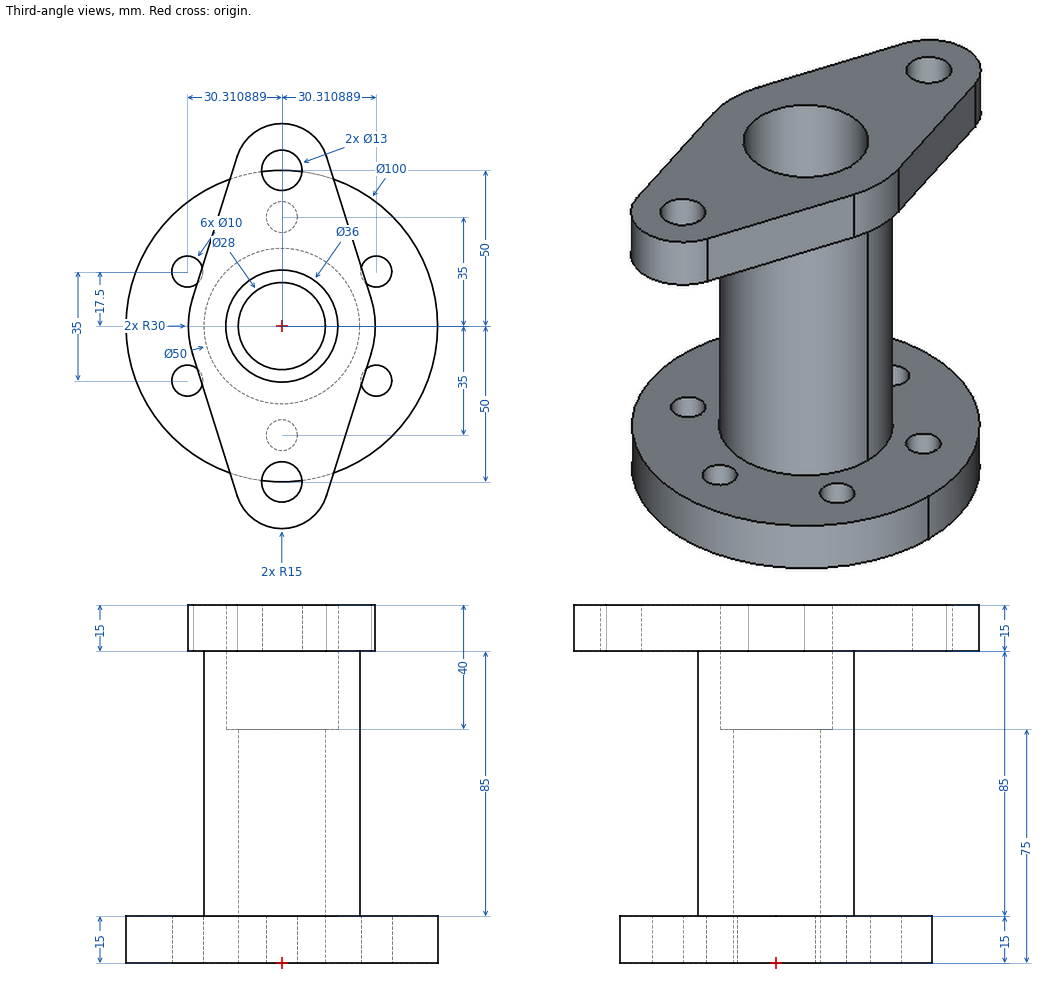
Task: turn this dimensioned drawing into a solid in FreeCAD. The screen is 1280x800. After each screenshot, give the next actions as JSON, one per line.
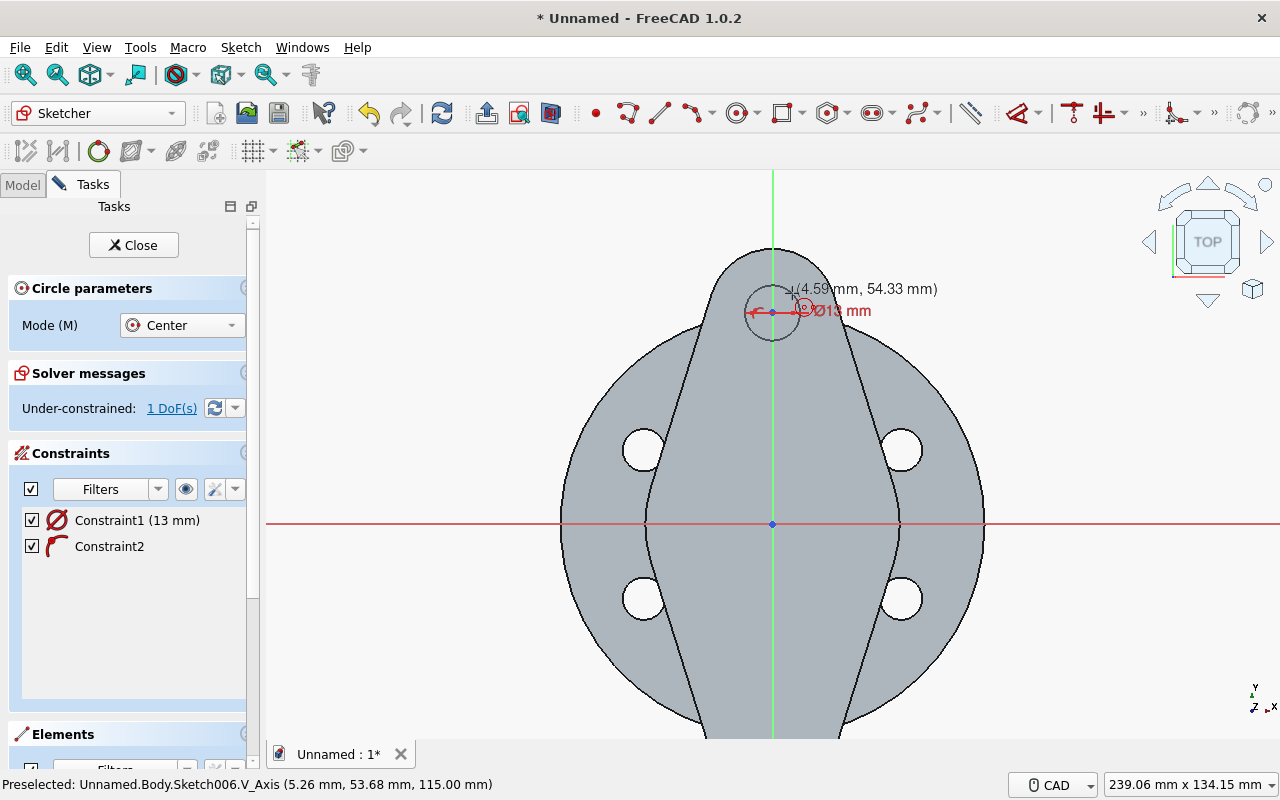
{"action": "scroll", "coordinate": [397, 198], "scroll_direction": "down", "scroll_amount": 1}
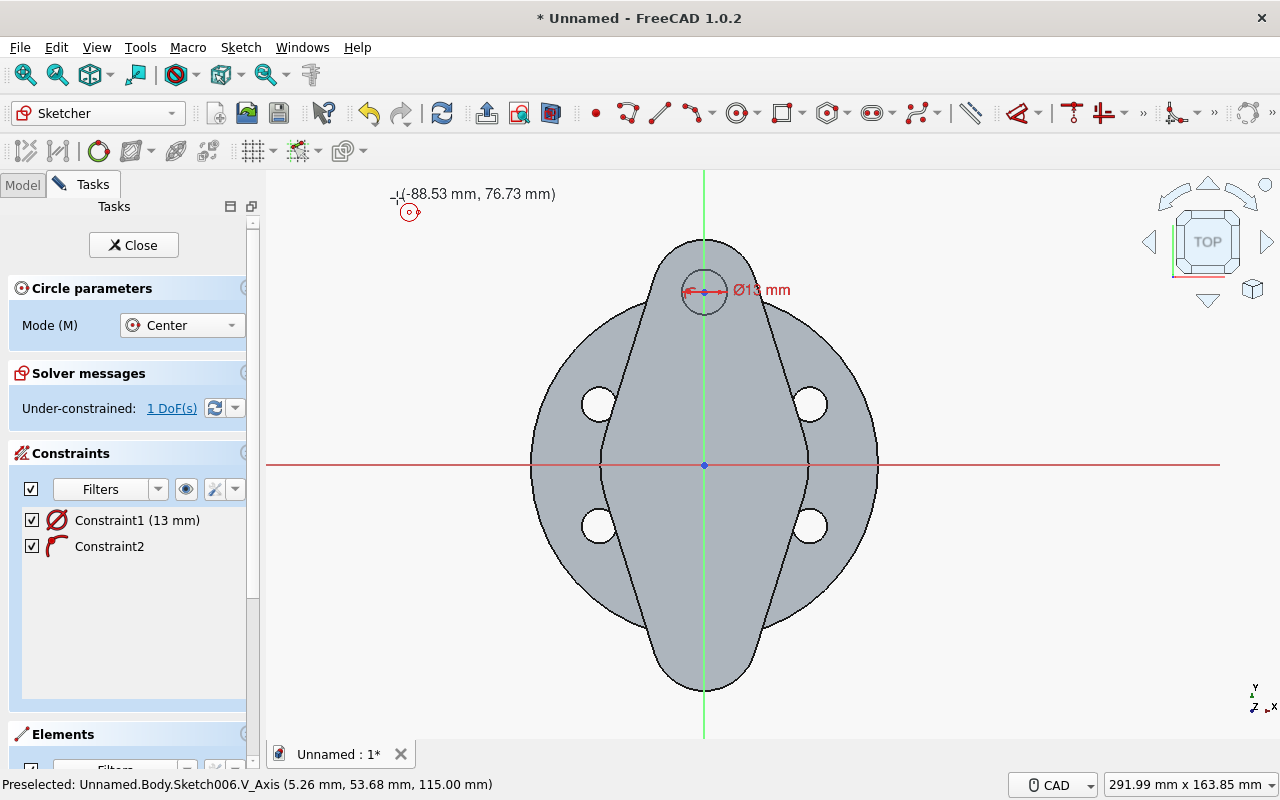
{"action": "left_click", "coordinate": [704, 639]}
{"action": "mouse_move", "coordinate": [720, 623]}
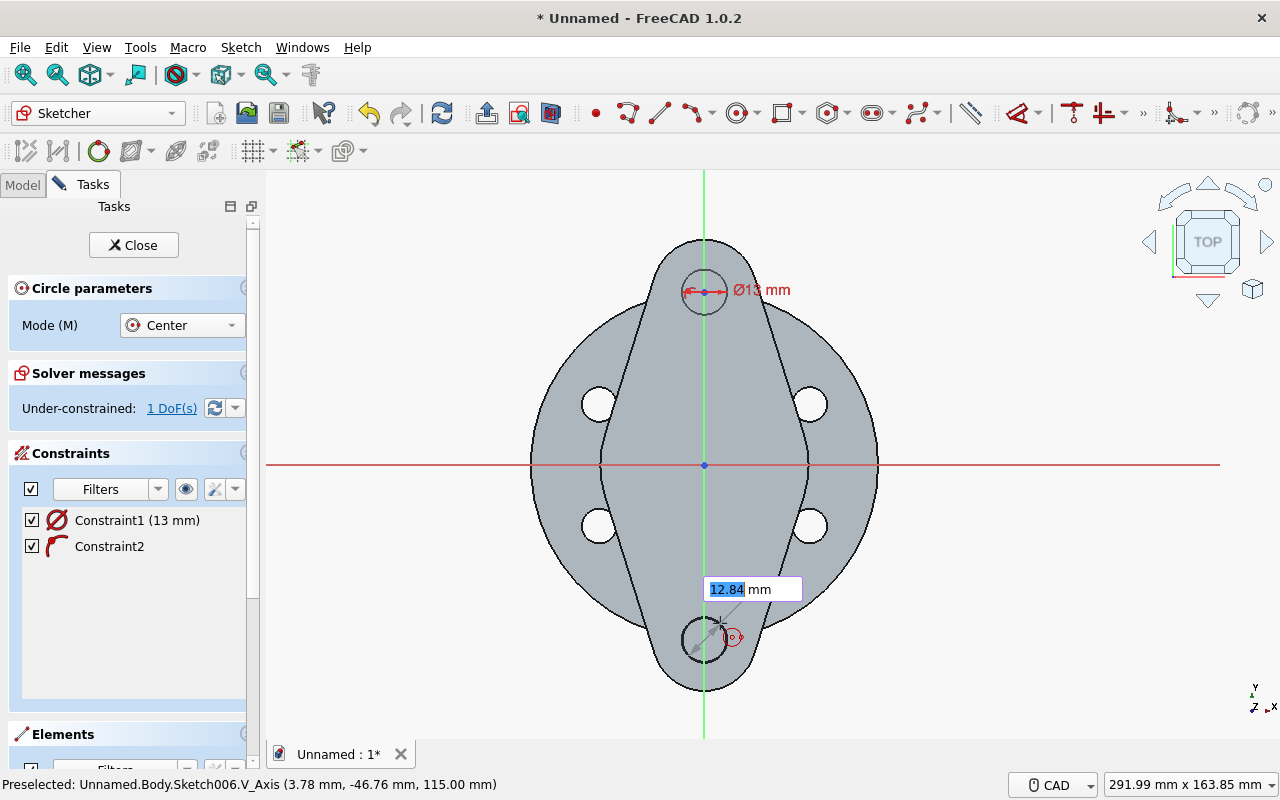
{"action": "type", "text": "13"}
{"action": "key", "text": "Return"}
{"action": "key", "text": "Escape"}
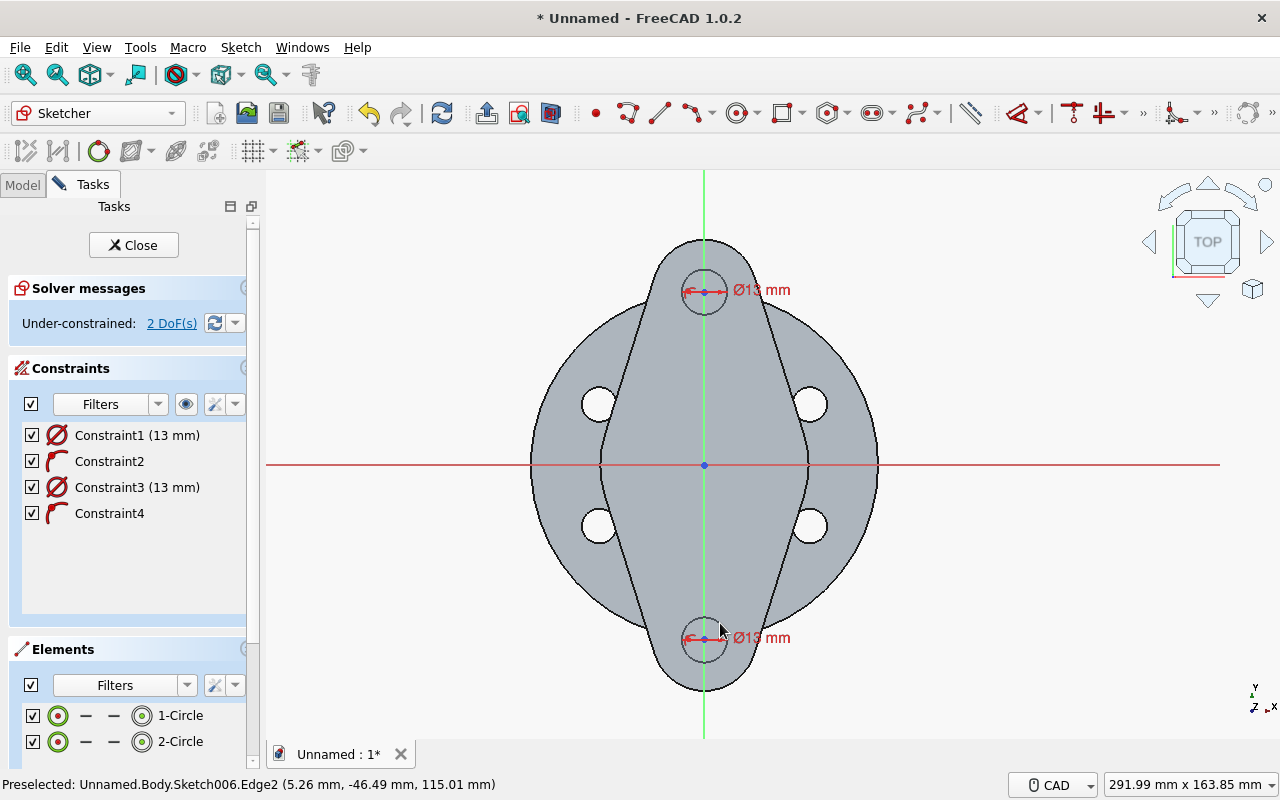
{"action": "left_click", "coordinate": [704, 292]}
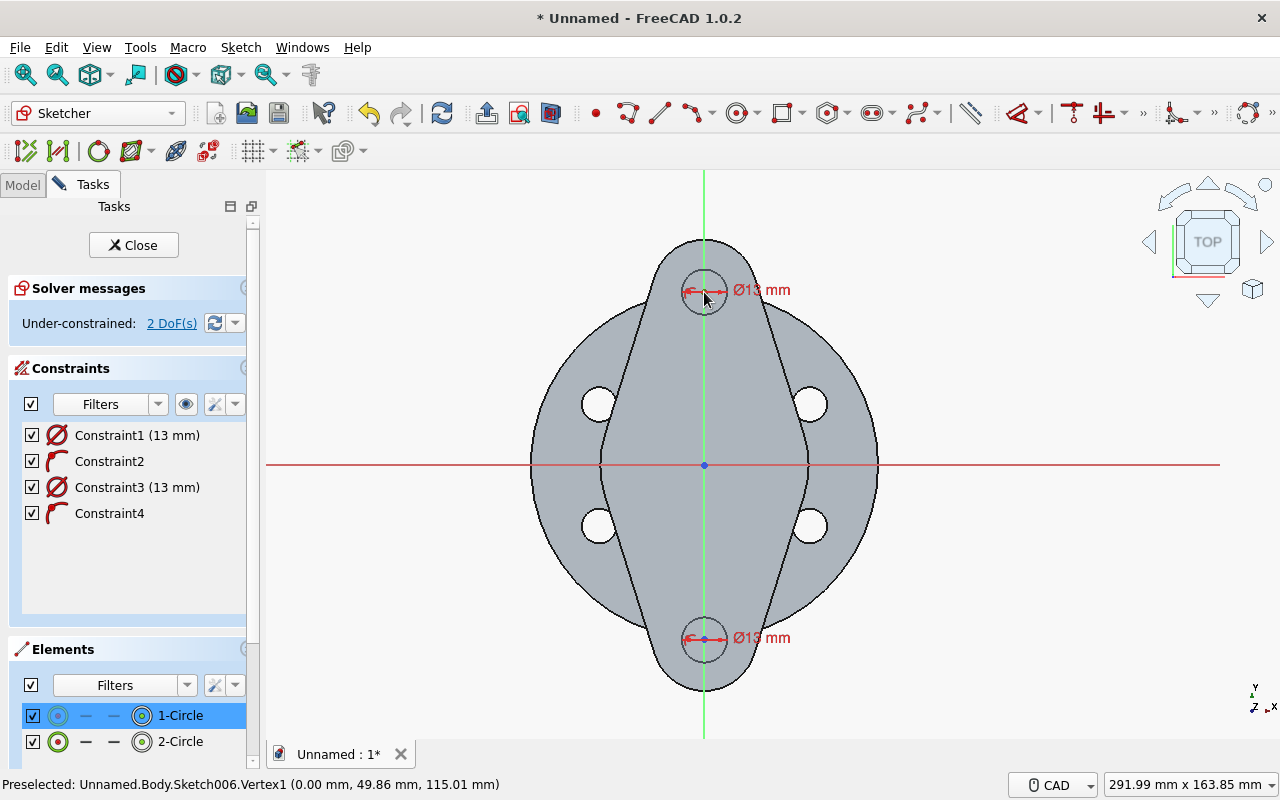
{"action": "key", "text": "i"}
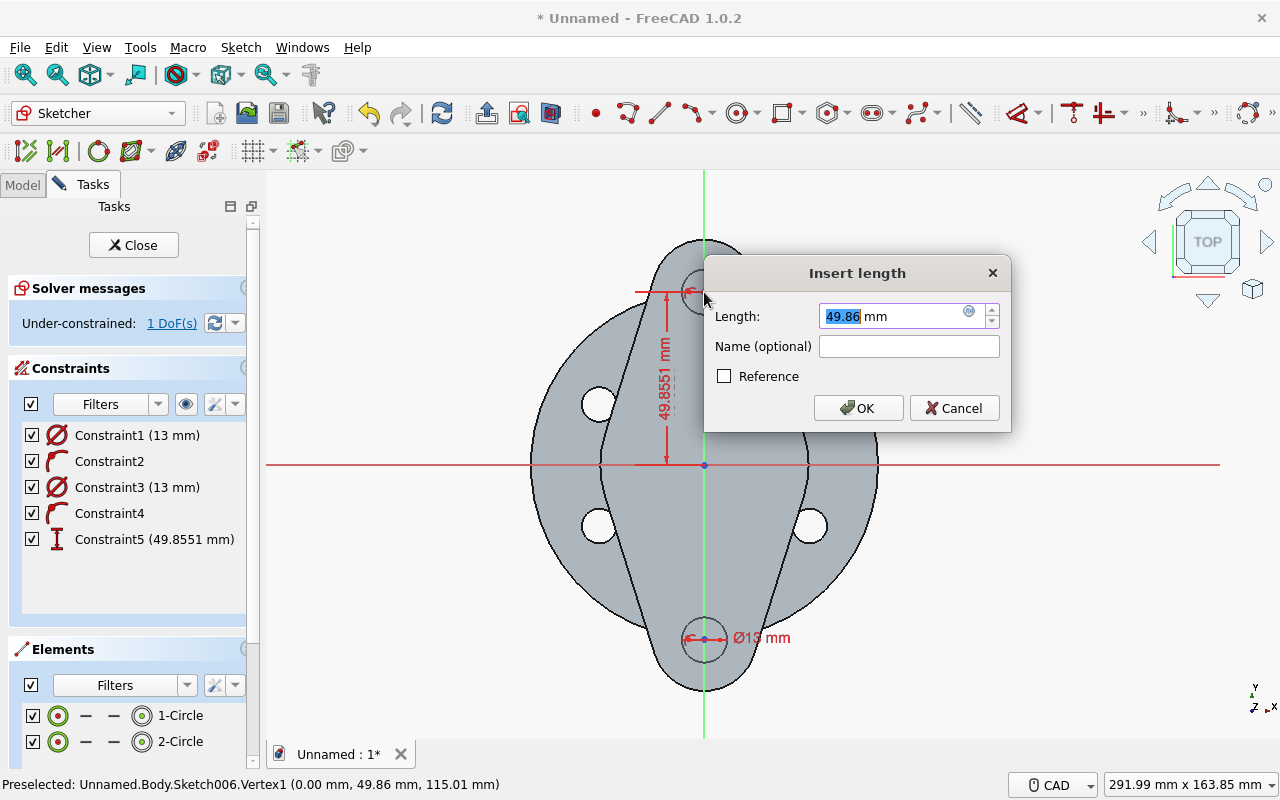
{"action": "type", "text": "50"}
{"action": "key", "text": "Return"}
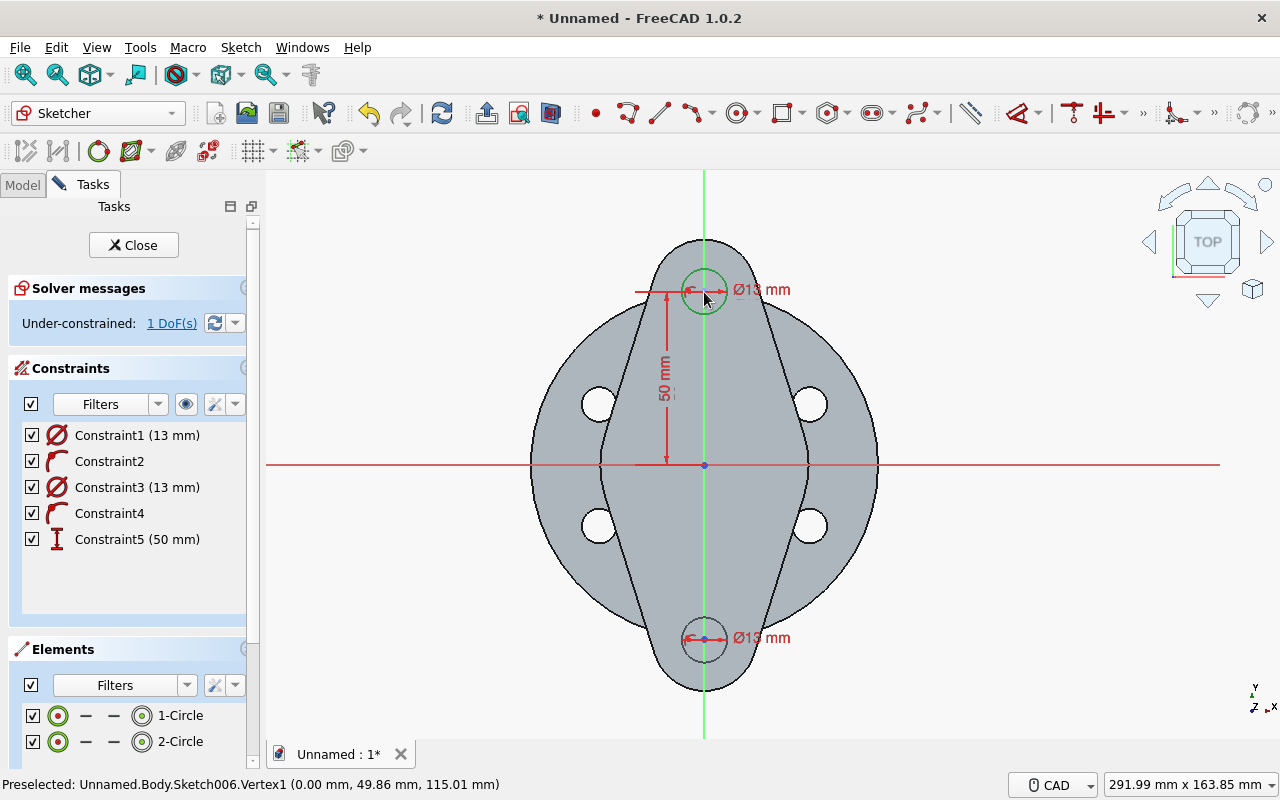
{"action": "left_click", "coordinate": [704, 640]}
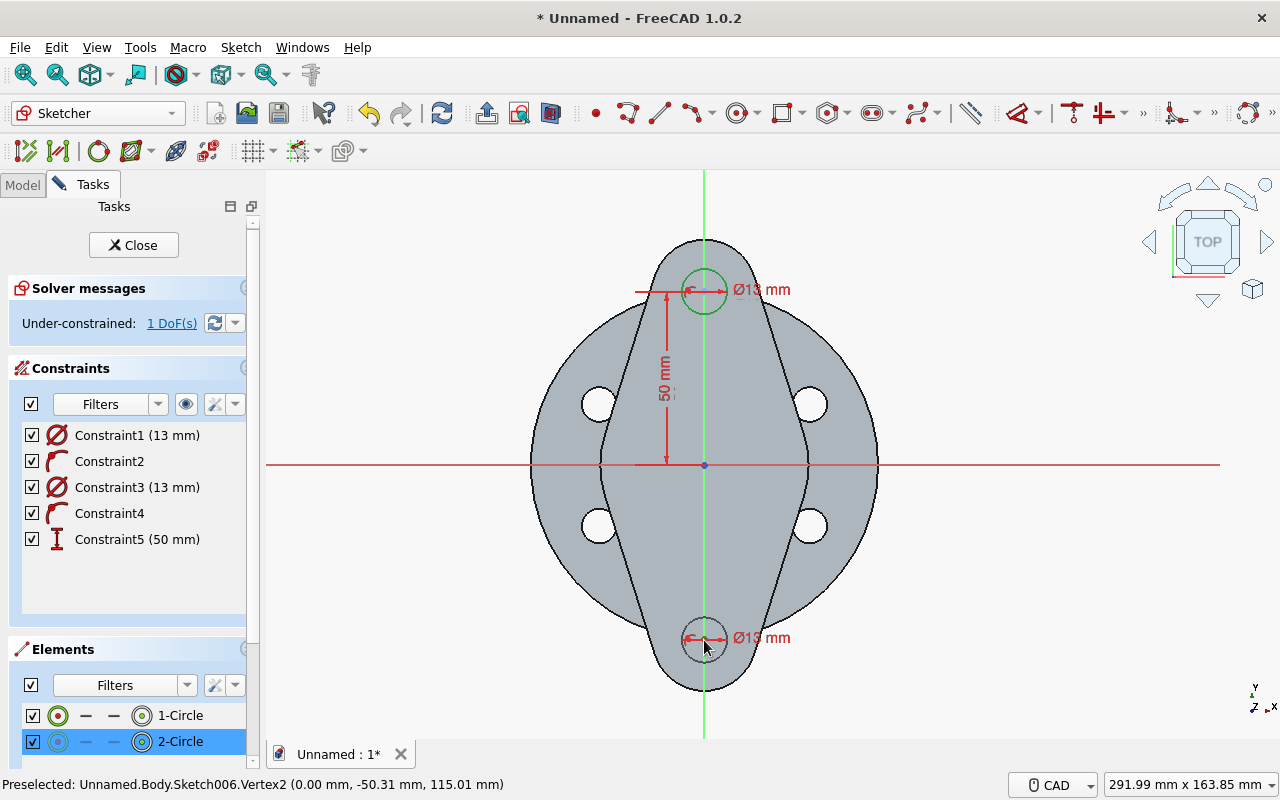
{"action": "key", "text": "i"}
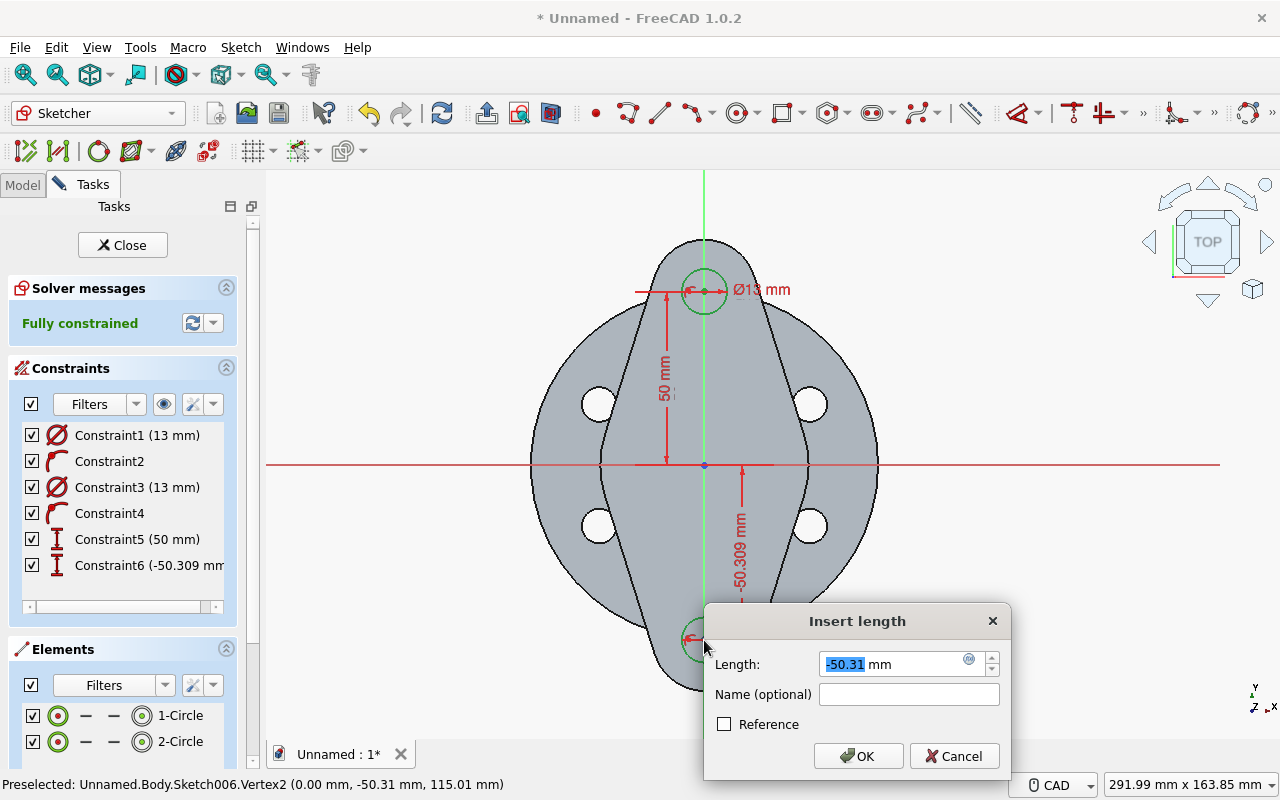
{"action": "type", "text": "-50"}
{"action": "key", "text": "Return"}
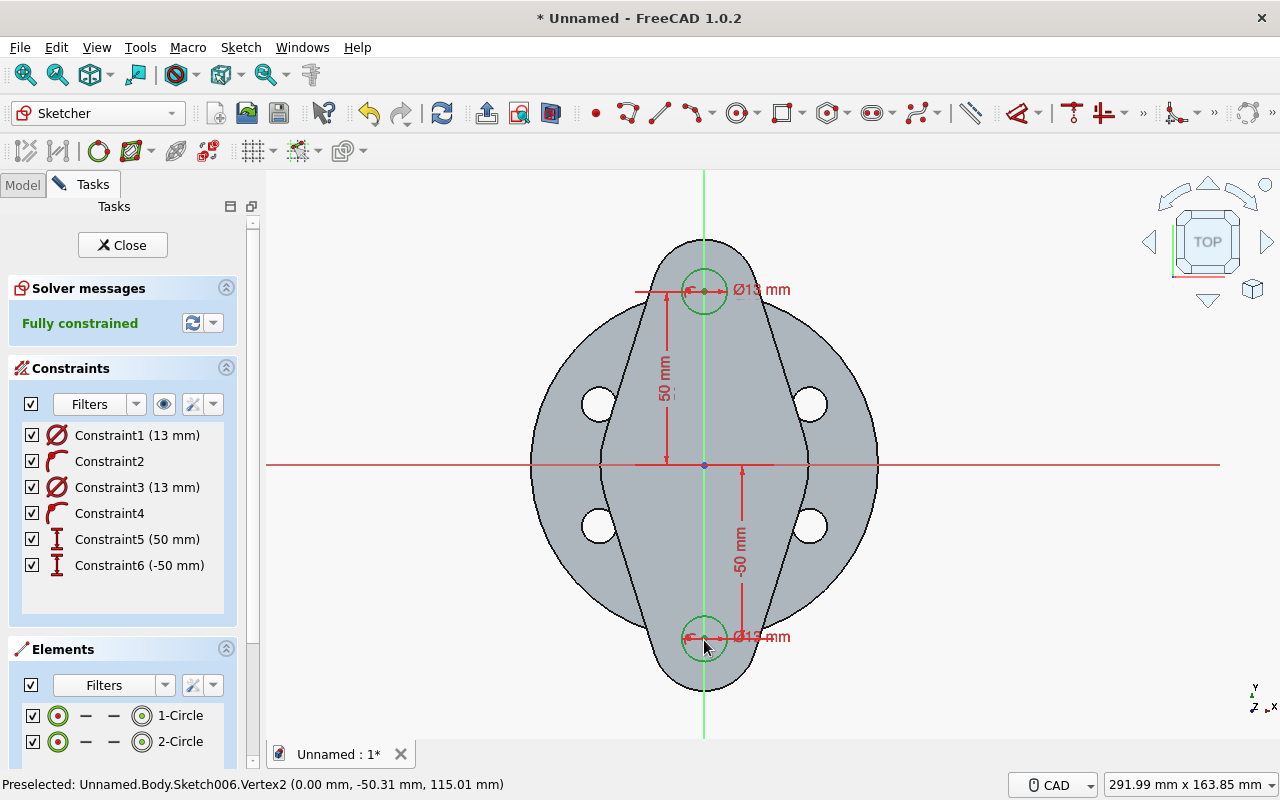
{"action": "left_click", "coordinate": [123, 245]}